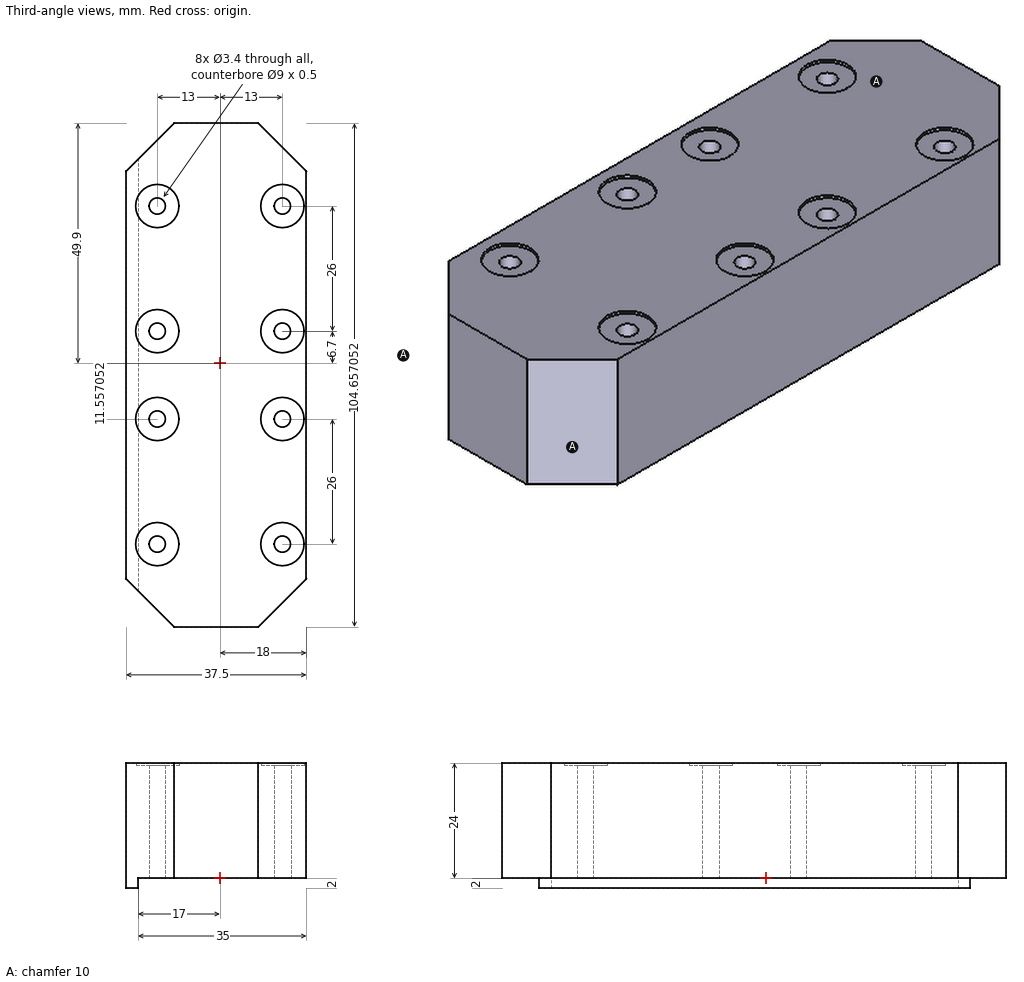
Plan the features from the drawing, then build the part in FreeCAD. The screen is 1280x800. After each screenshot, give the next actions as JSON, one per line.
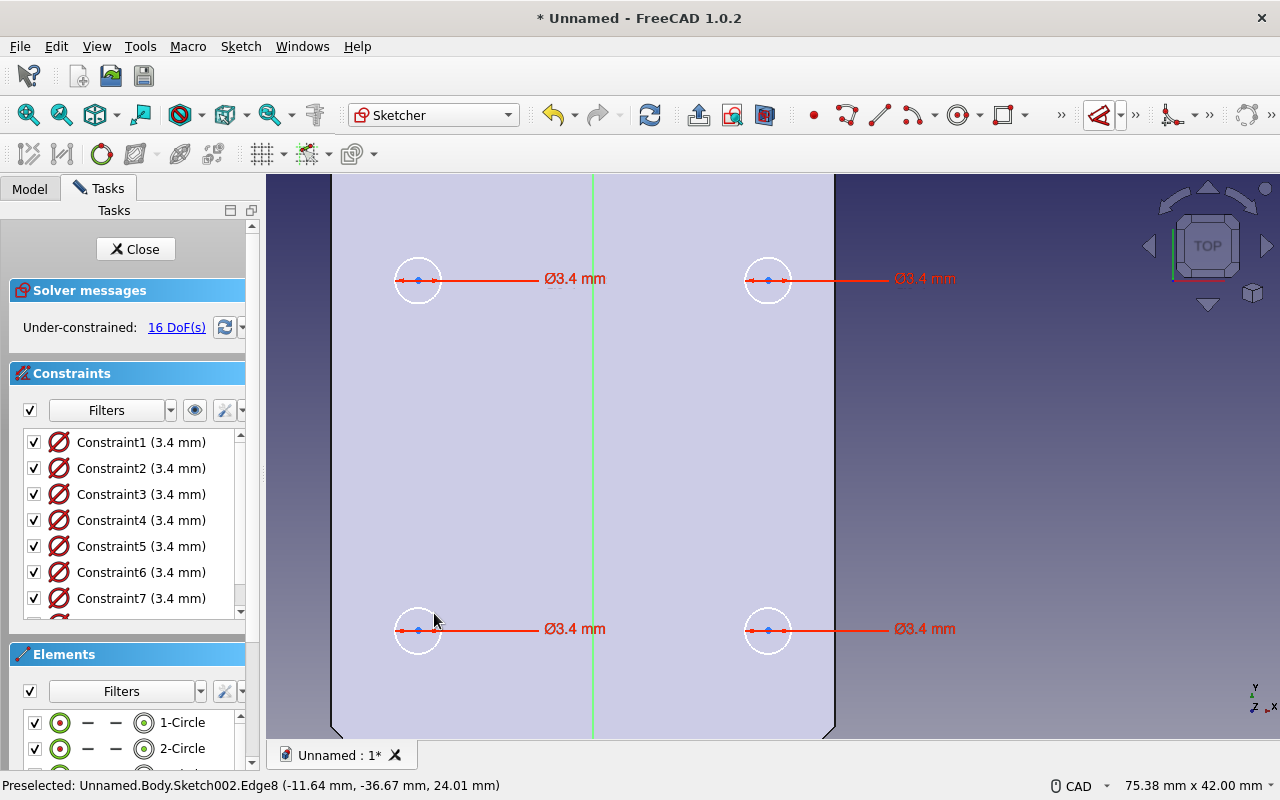
{"action": "scroll", "coordinate": [769, 631], "scroll_direction": "down", "scroll_amount": 5}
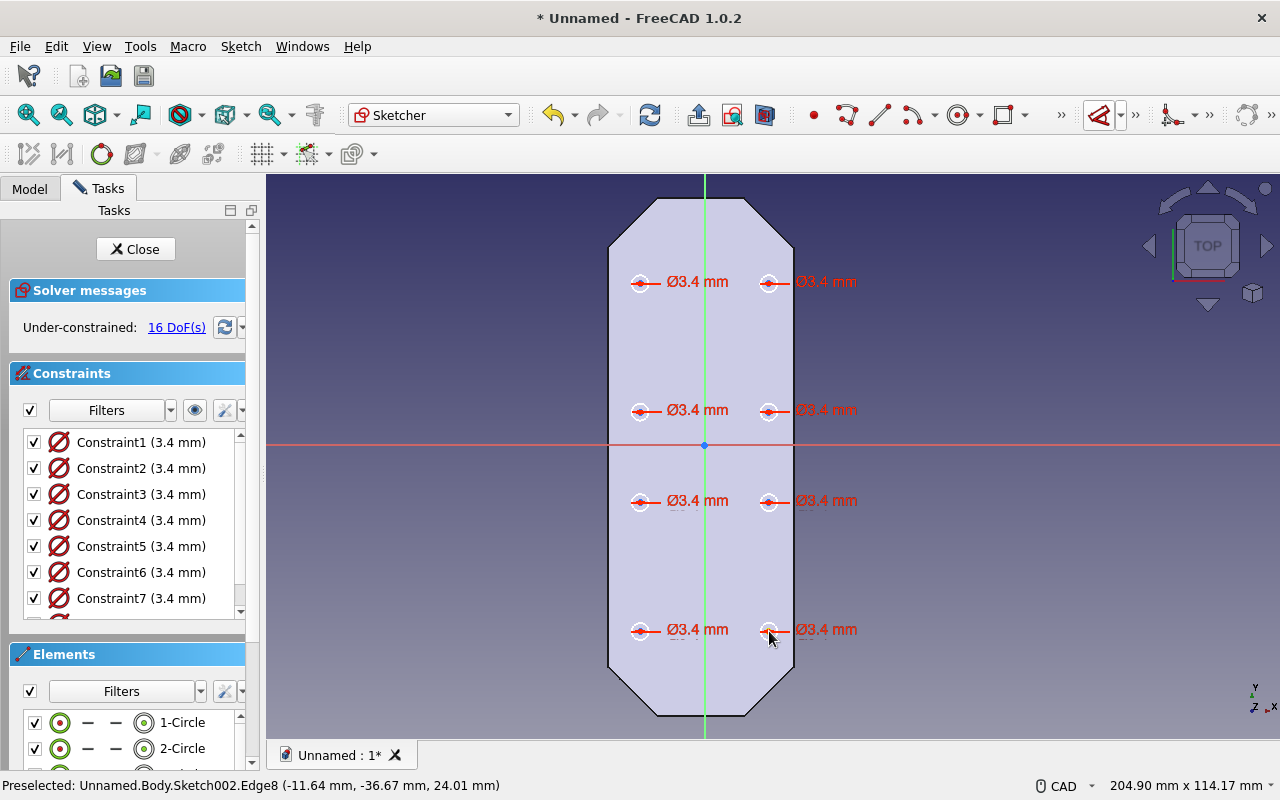
{"action": "left_click", "coordinate": [640, 284]}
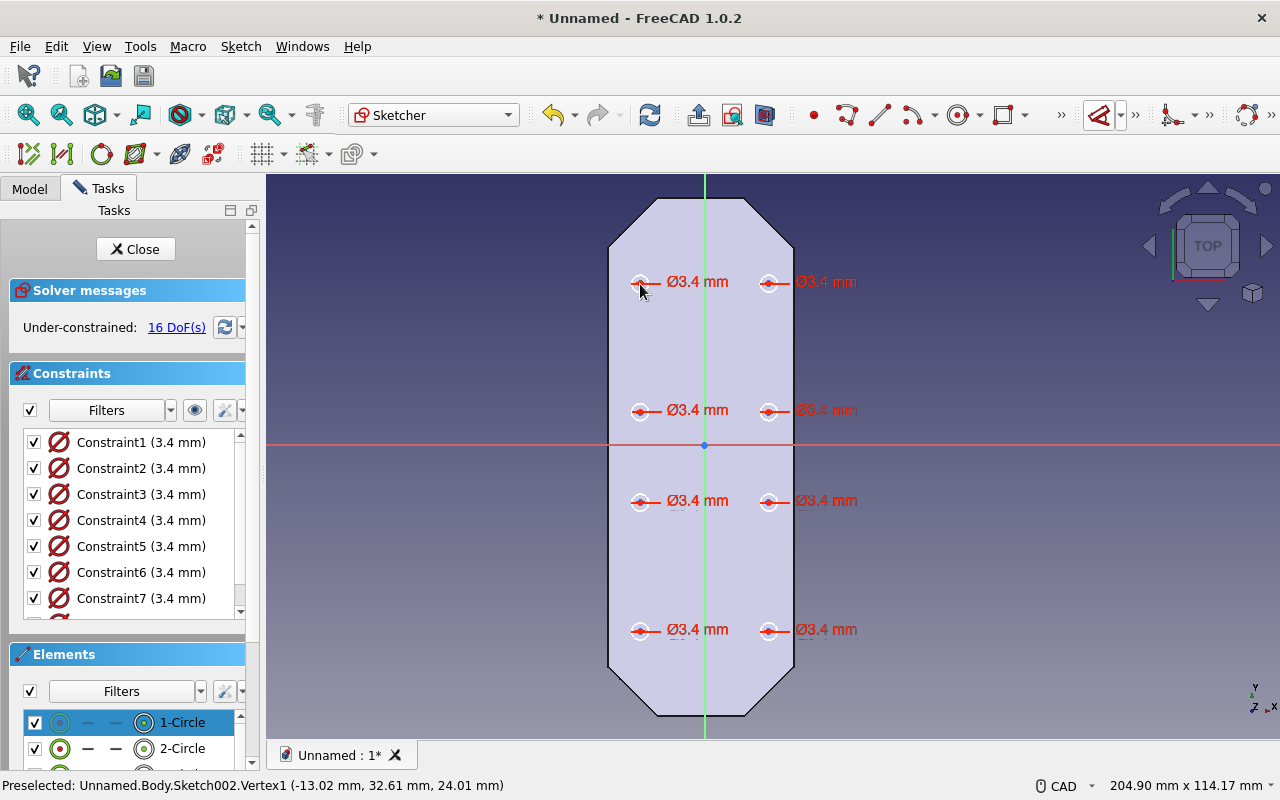
{"action": "left_click", "coordinate": [769, 284]}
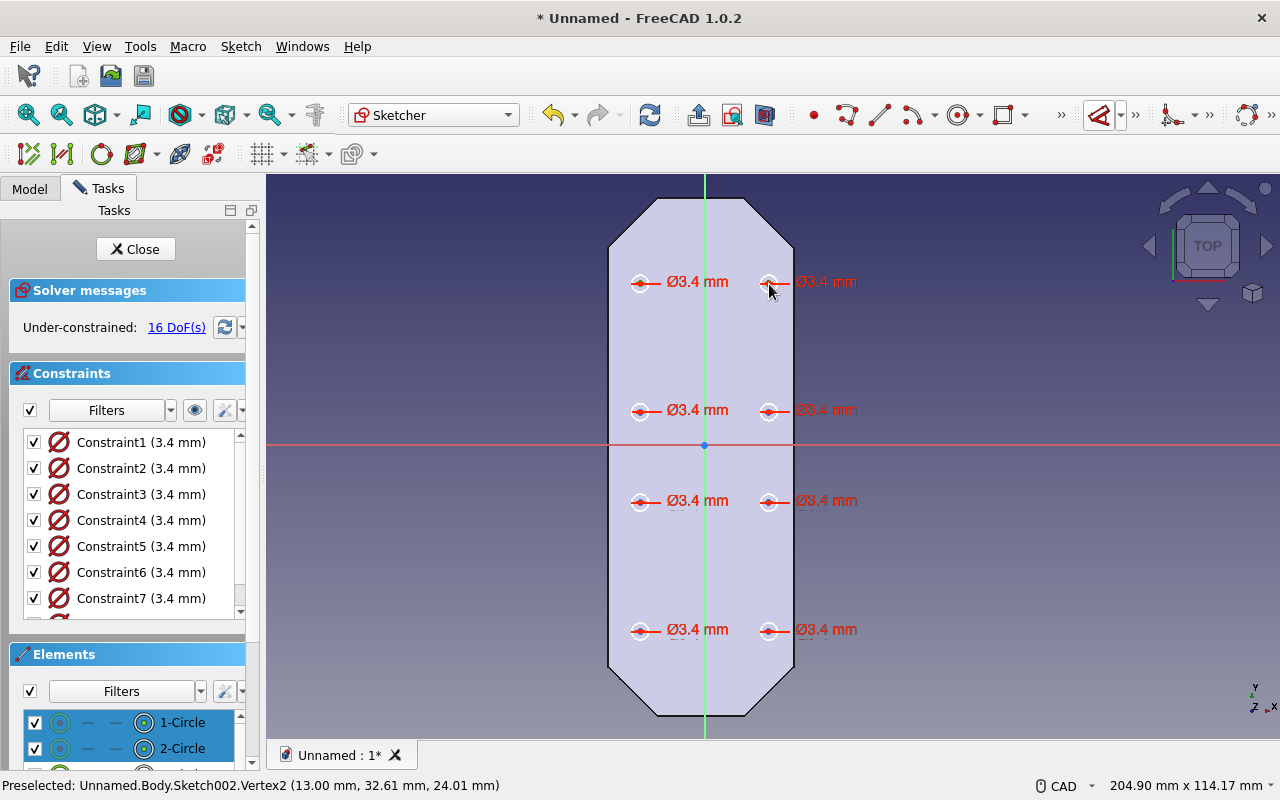
{"action": "key", "text": "h"}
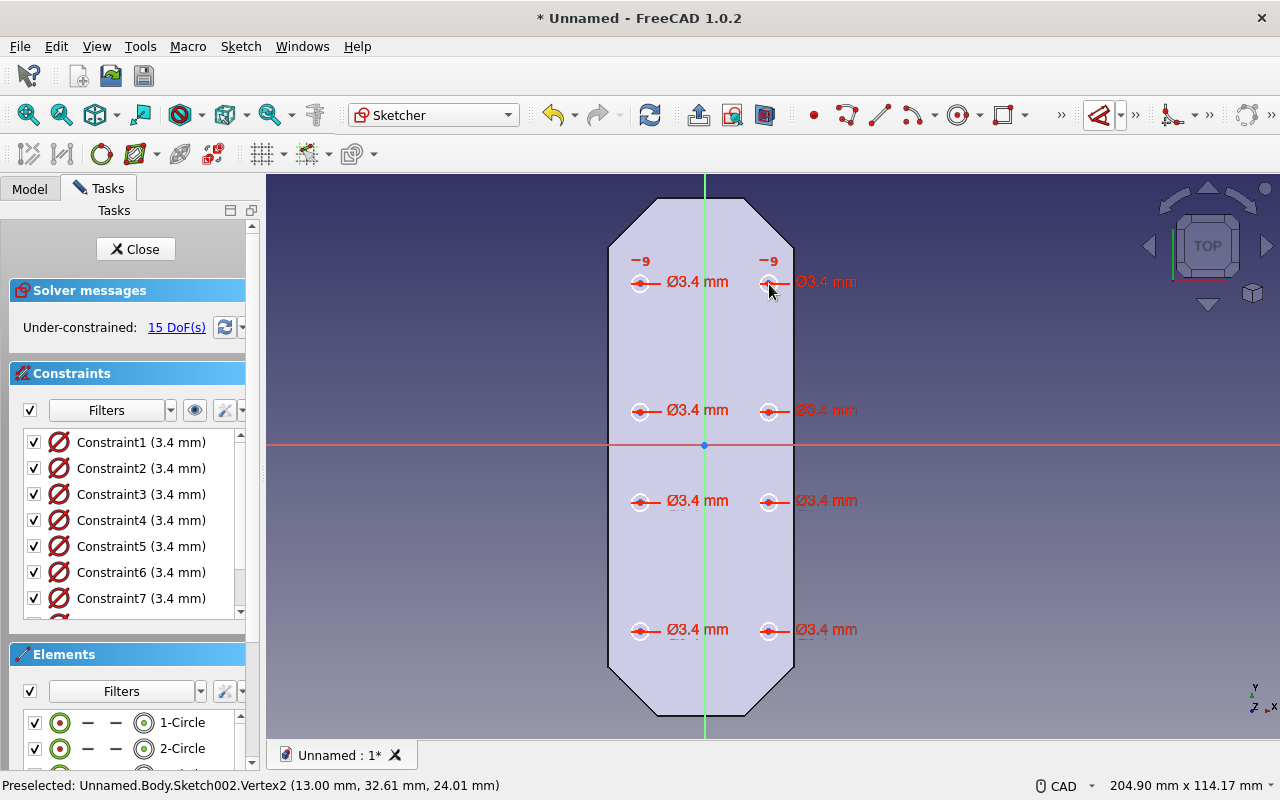
{"action": "left_click", "coordinate": [769, 284]}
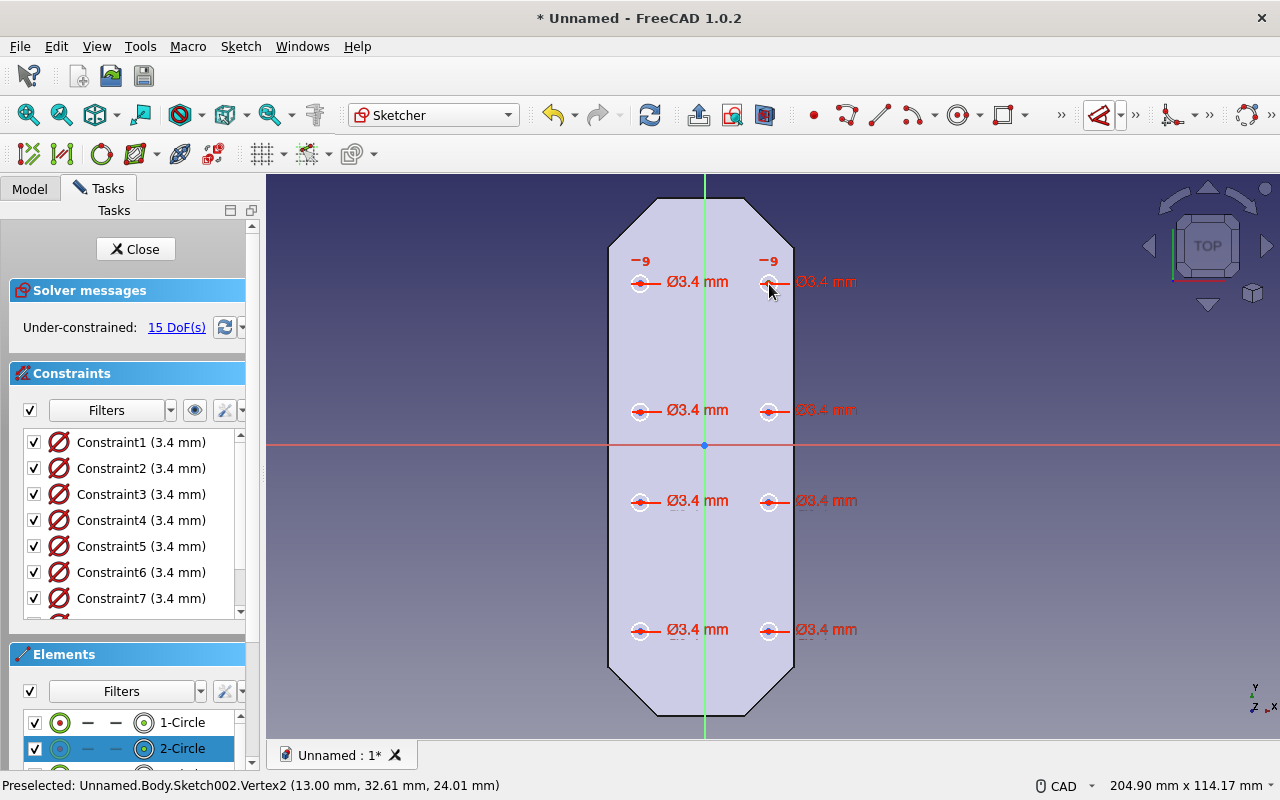
{"action": "left_click", "coordinate": [769, 412]}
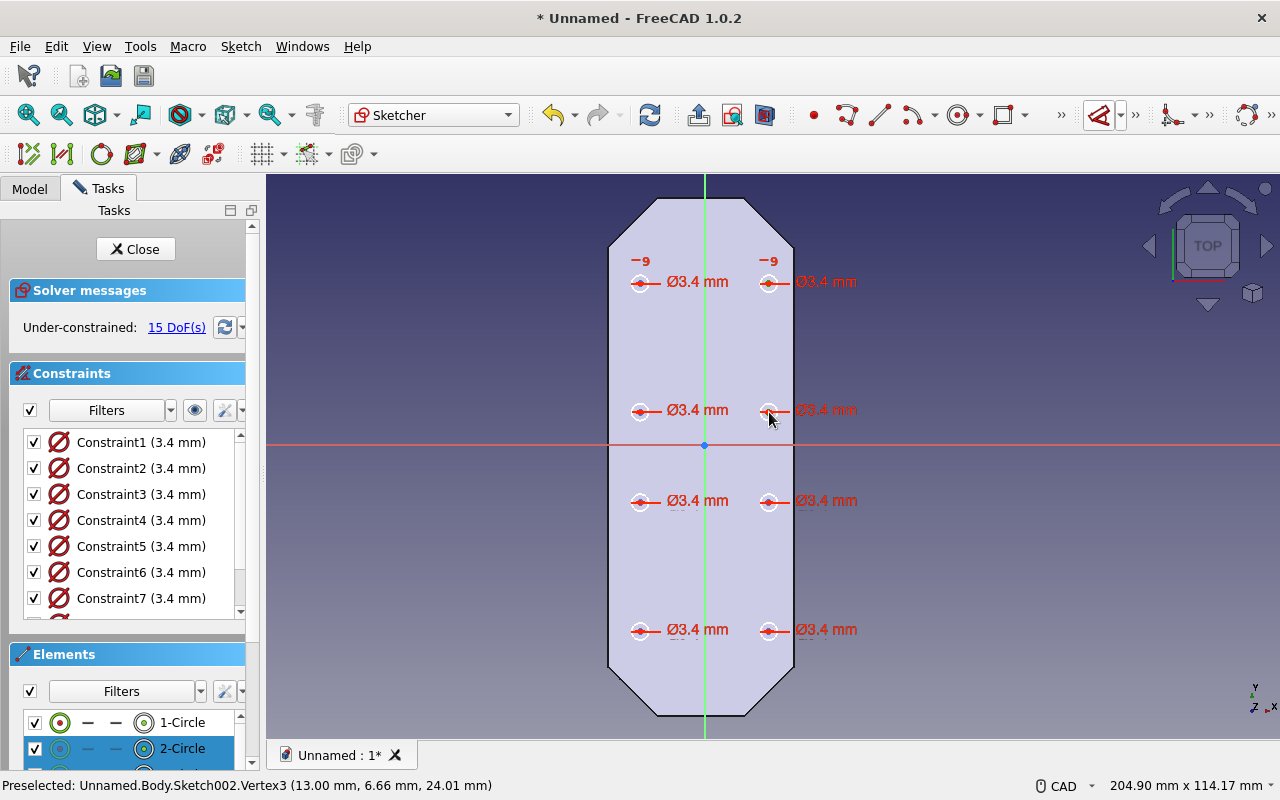
{"action": "key", "text": "v"}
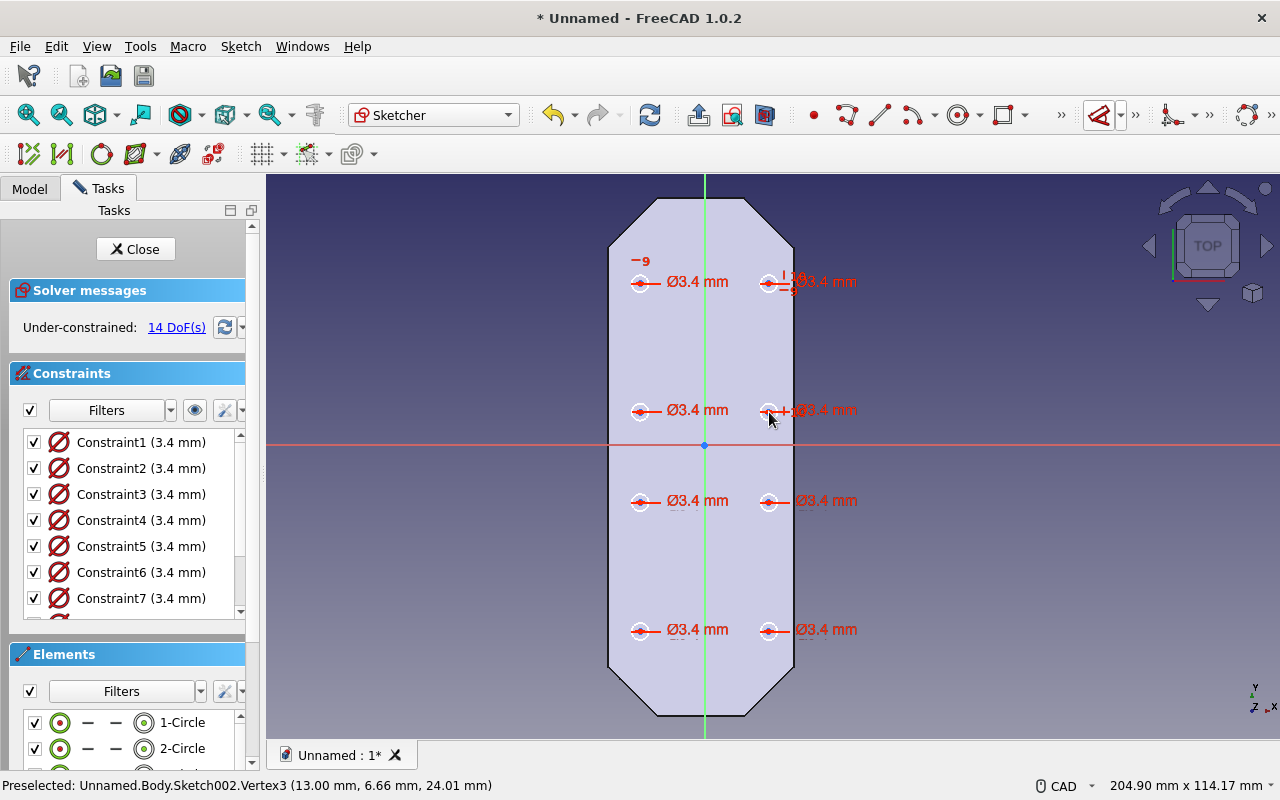
{"action": "left_click", "coordinate": [640, 284]}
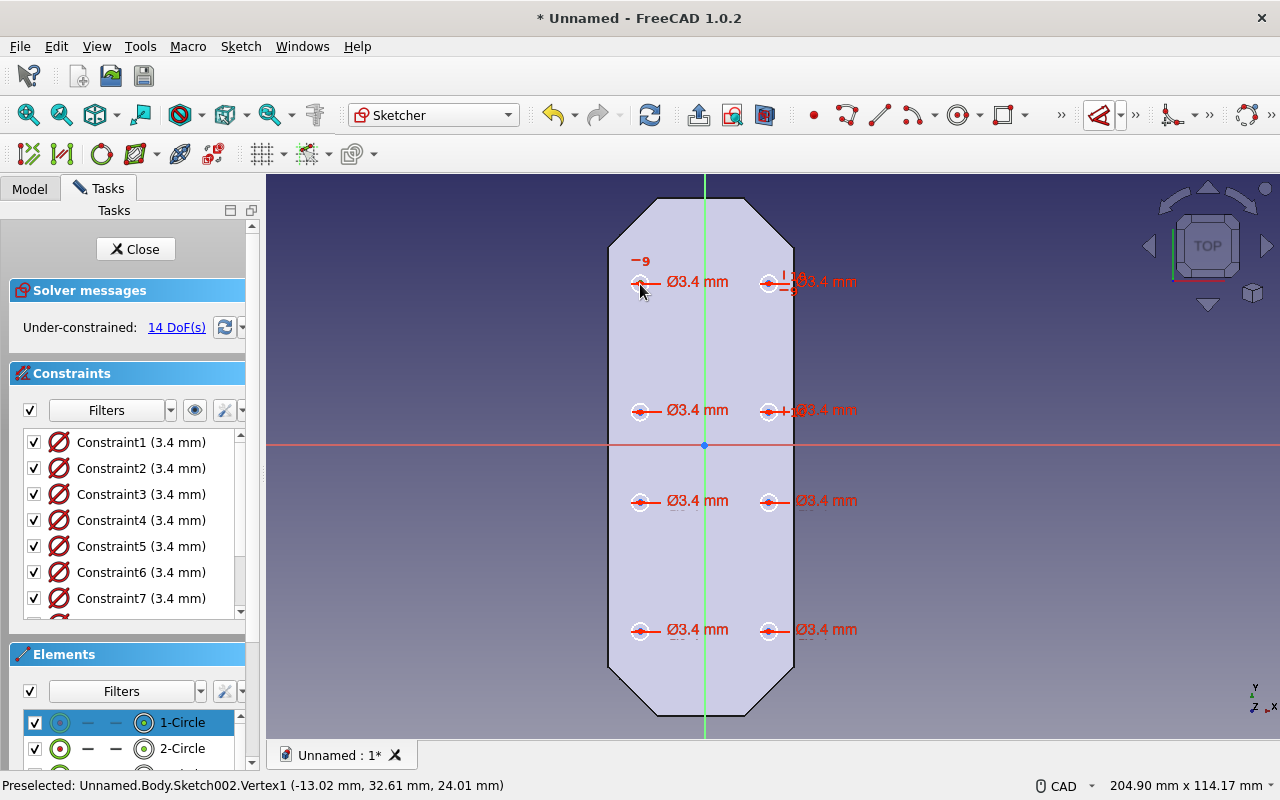
{"action": "left_click", "coordinate": [640, 412]}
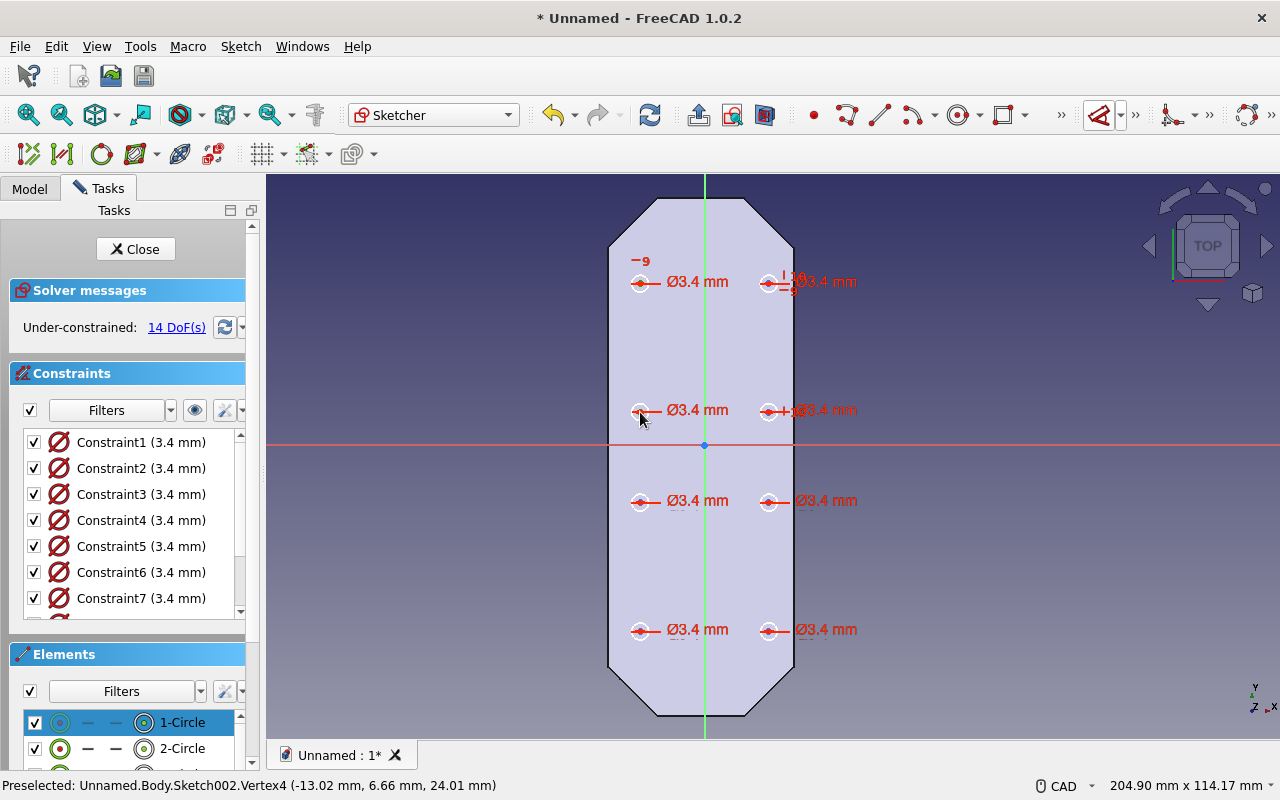
{"action": "key", "text": "v"}